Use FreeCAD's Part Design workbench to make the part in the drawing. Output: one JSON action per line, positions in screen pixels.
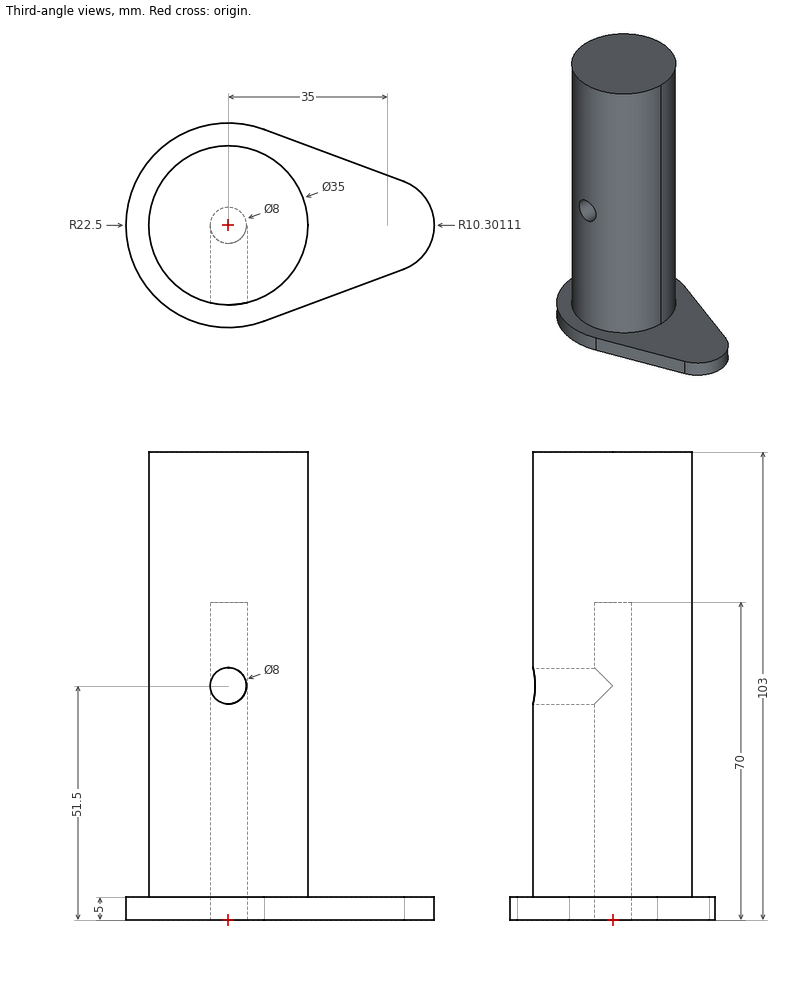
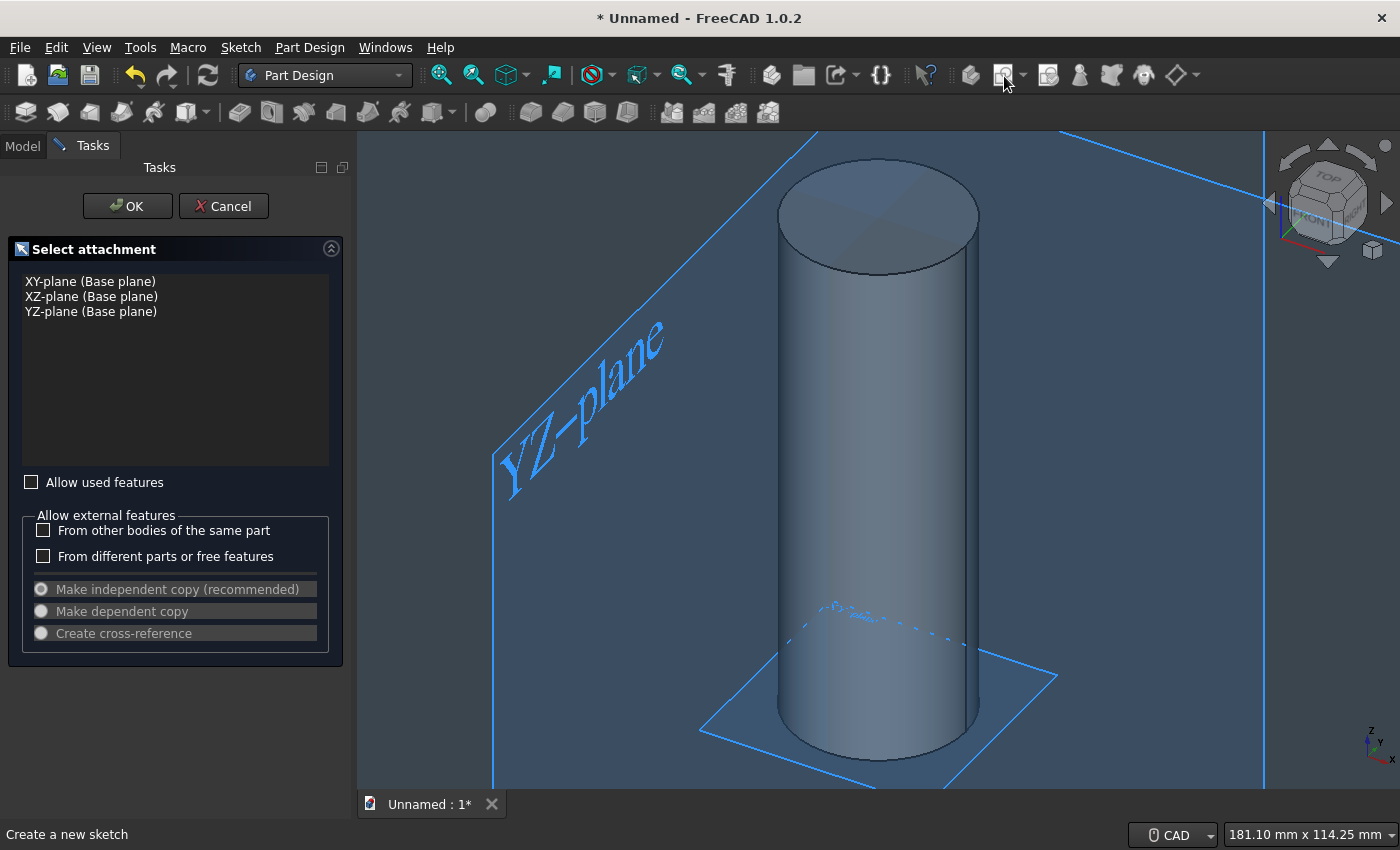
{"action": "left_click", "coordinate": [82, 282]}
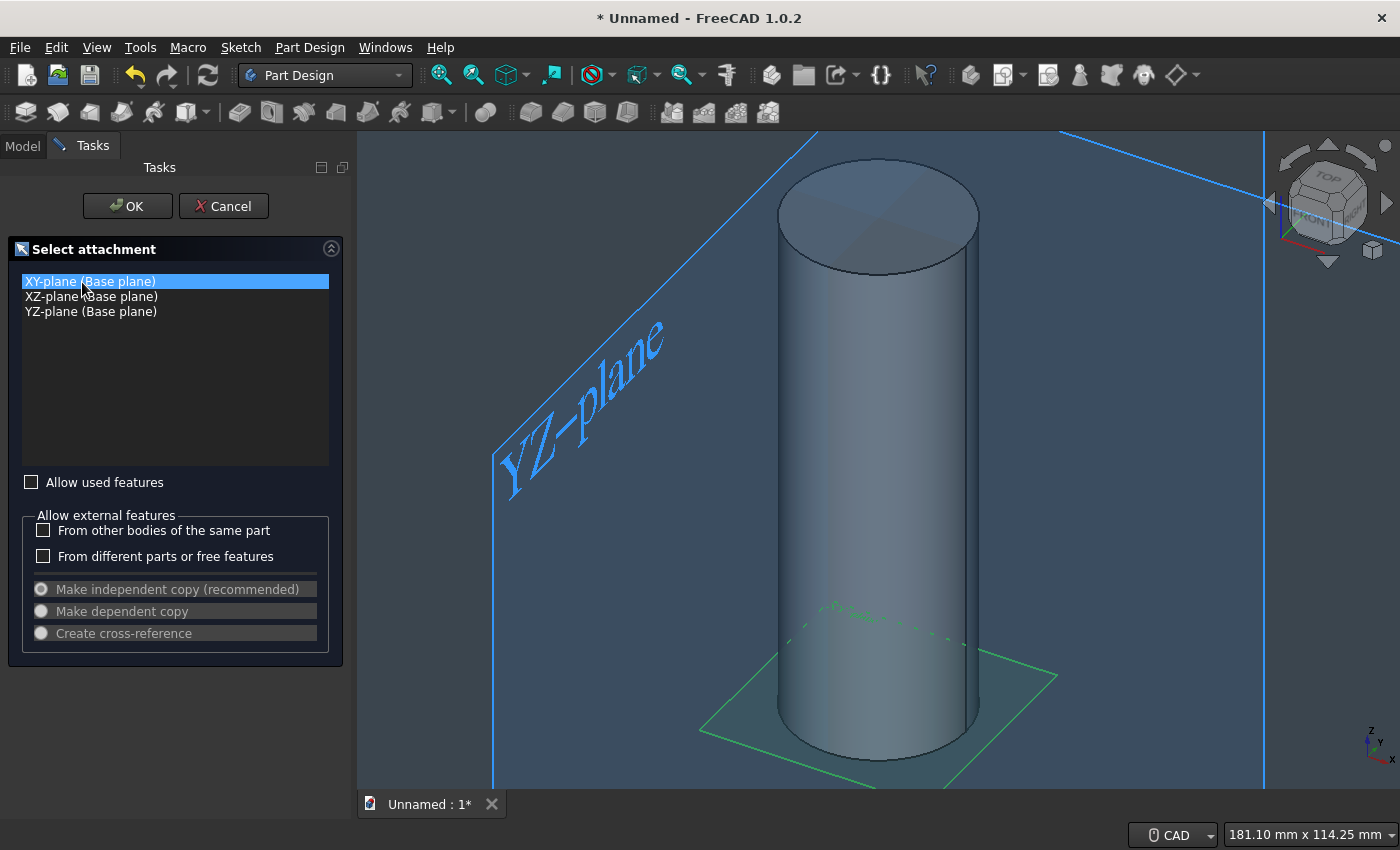
{"action": "left_click", "coordinate": [128, 206]}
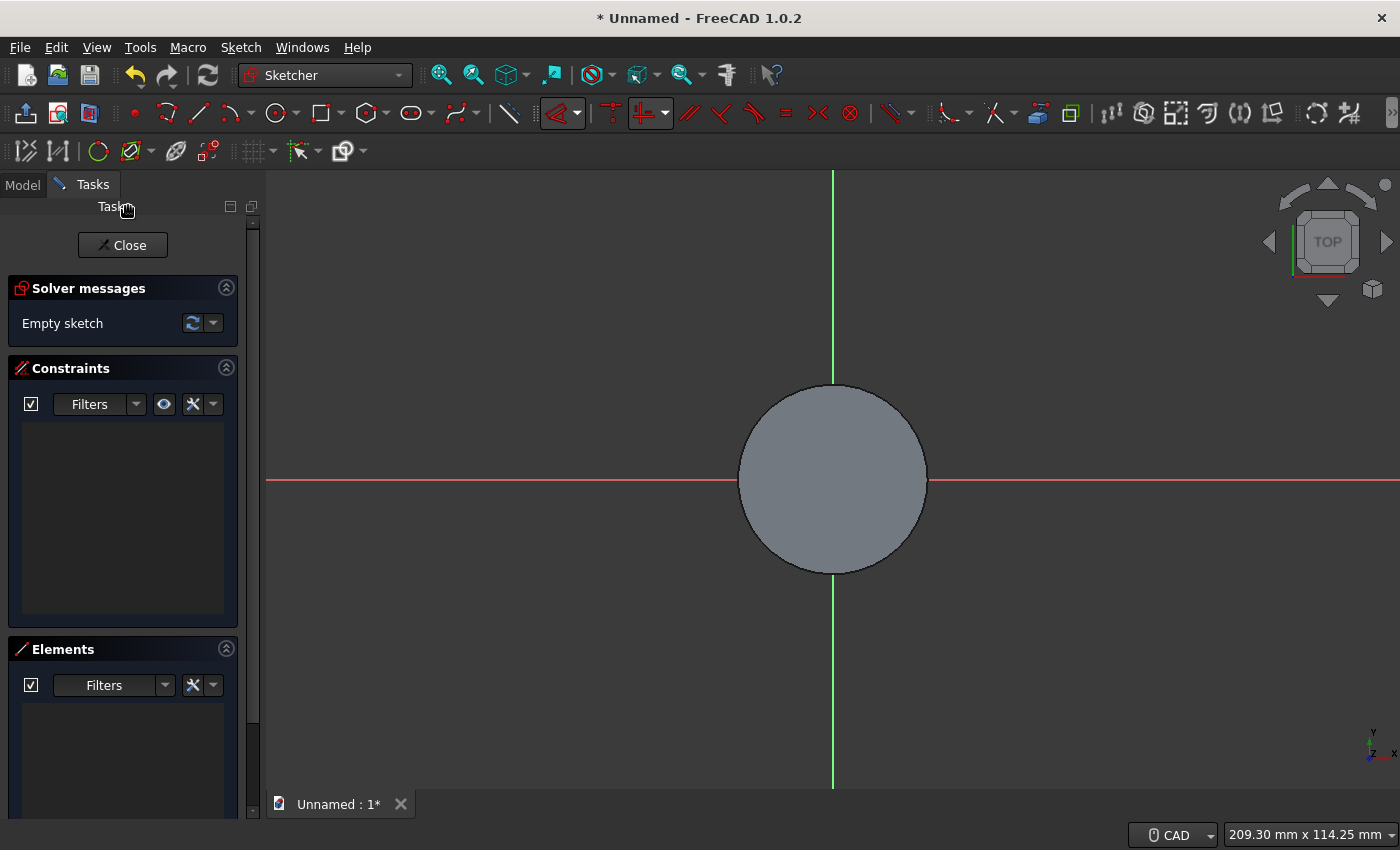
{"action": "left_click", "coordinate": [90, 114]}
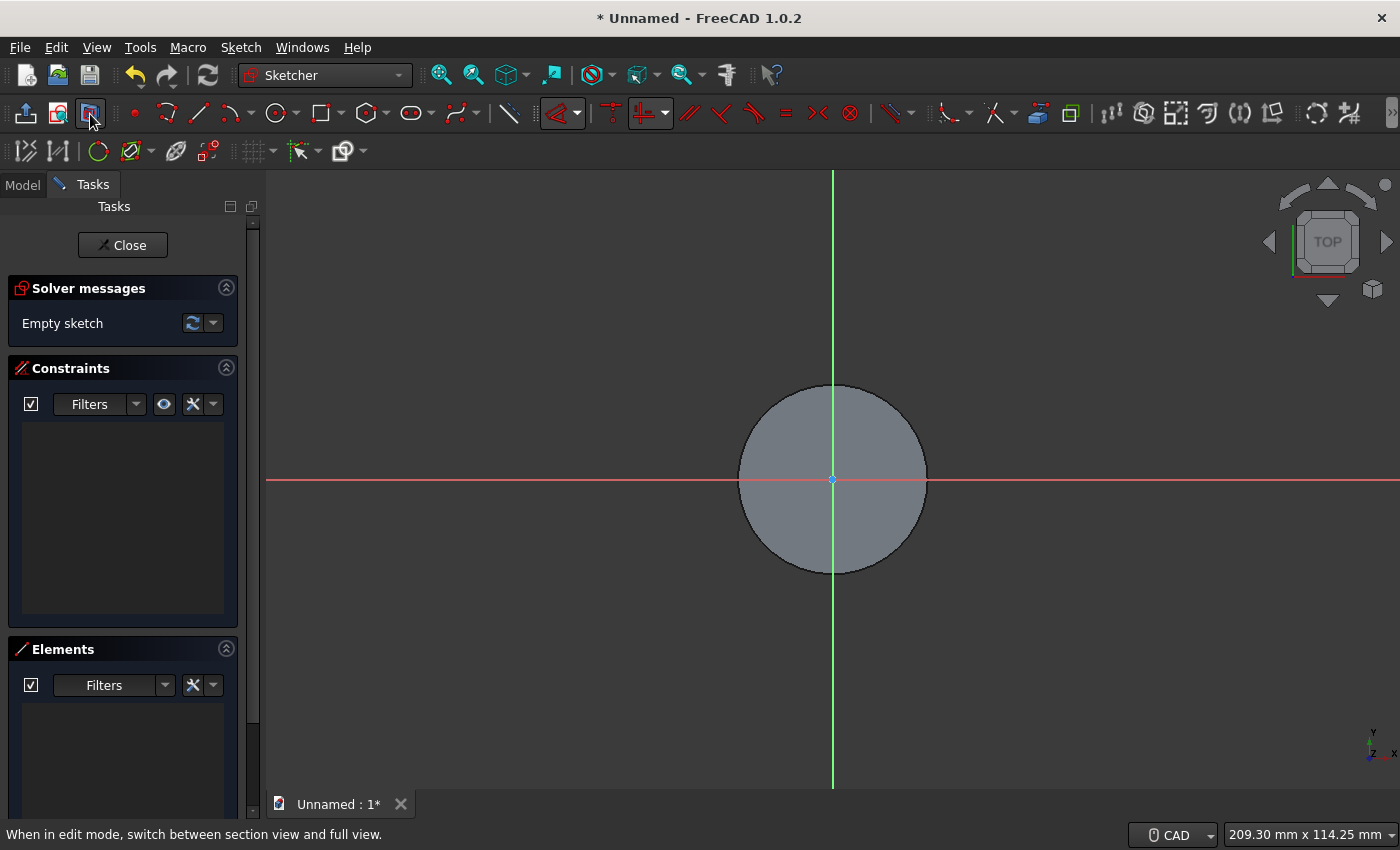
{"action": "scroll", "coordinate": [1053, 480], "scroll_direction": "up", "scroll_amount": 3}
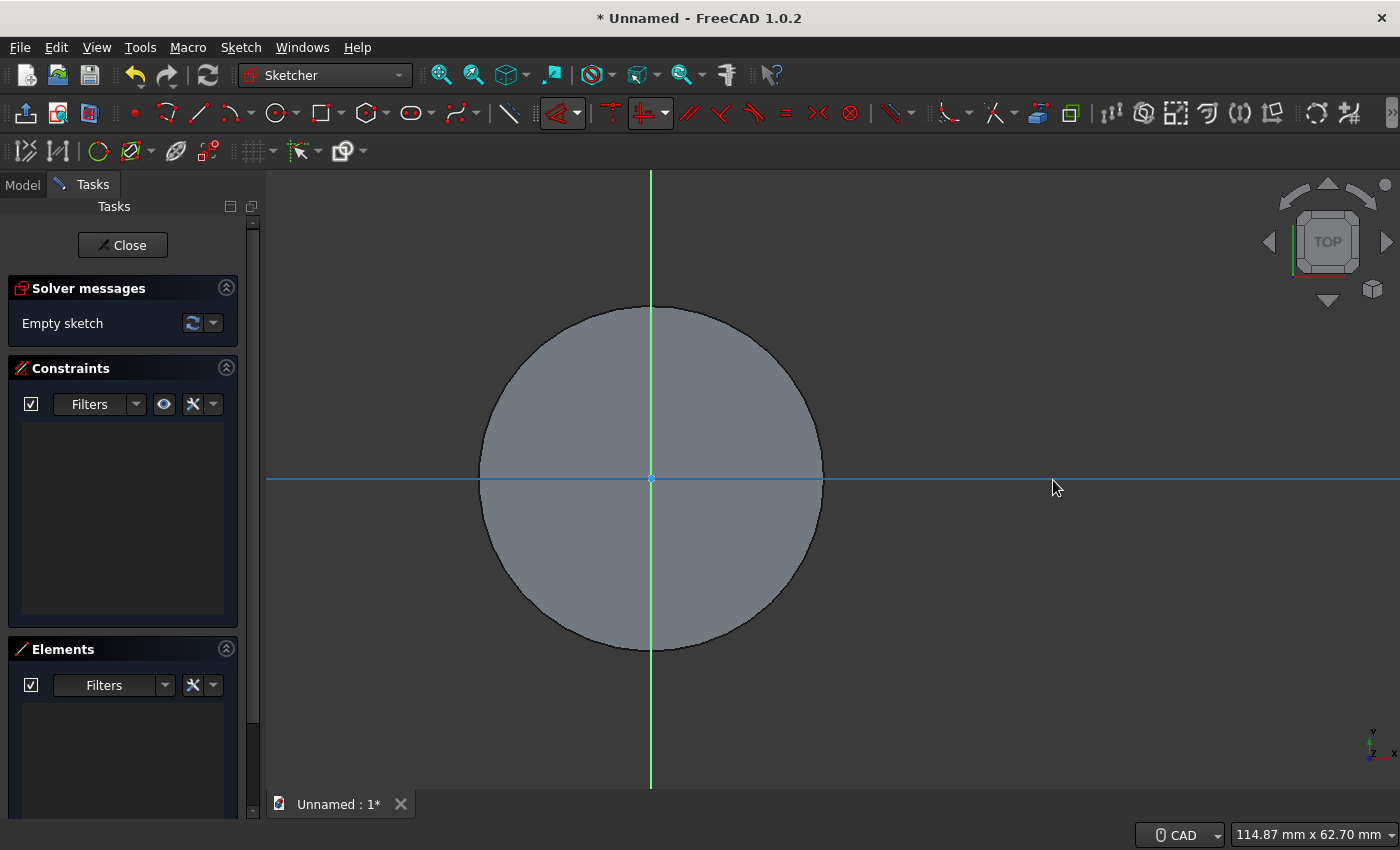
{"action": "left_click", "coordinate": [200, 114]}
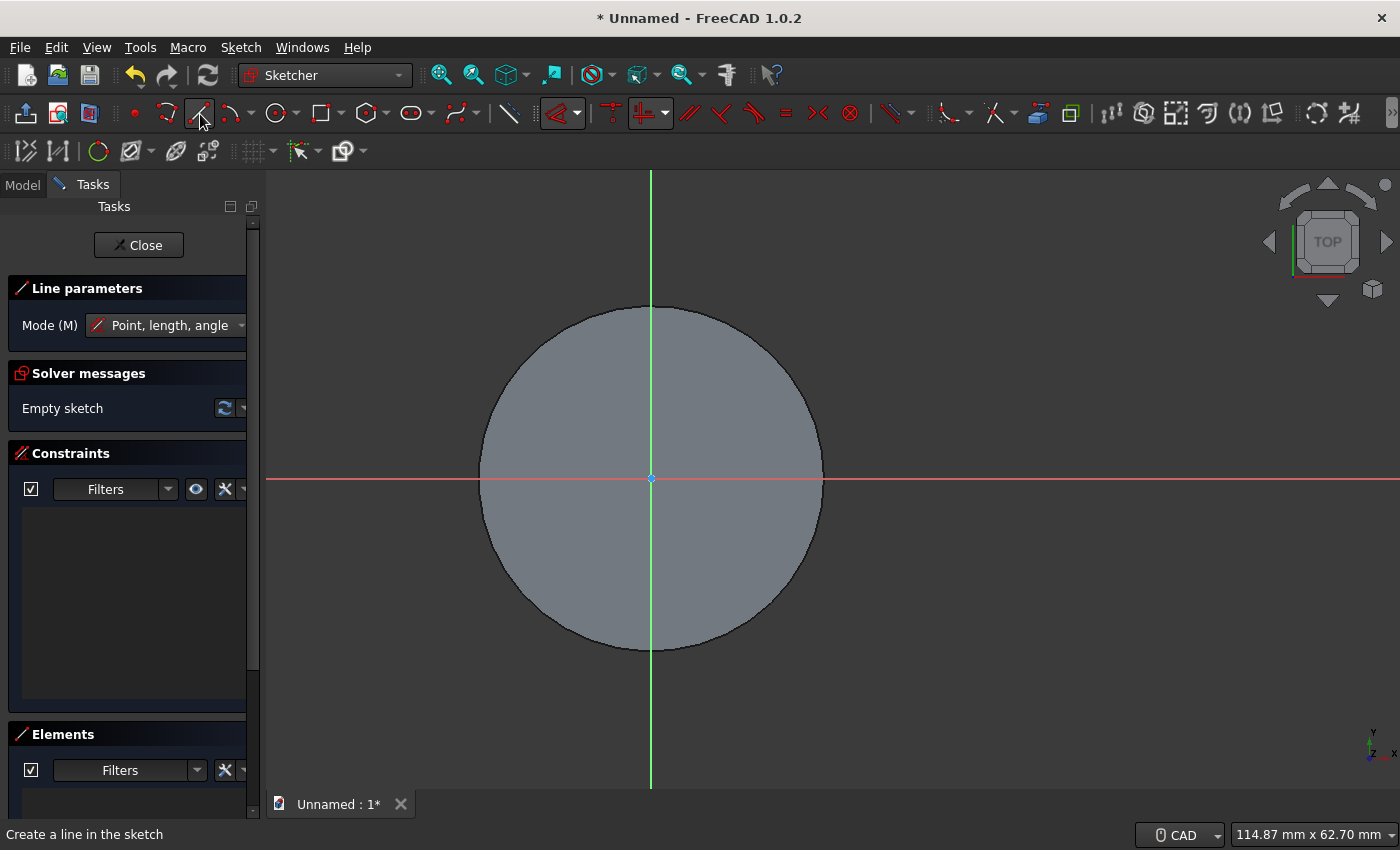
{"action": "left_click", "coordinate": [729, 270]}
{"action": "left_click", "coordinate": [1032, 383]}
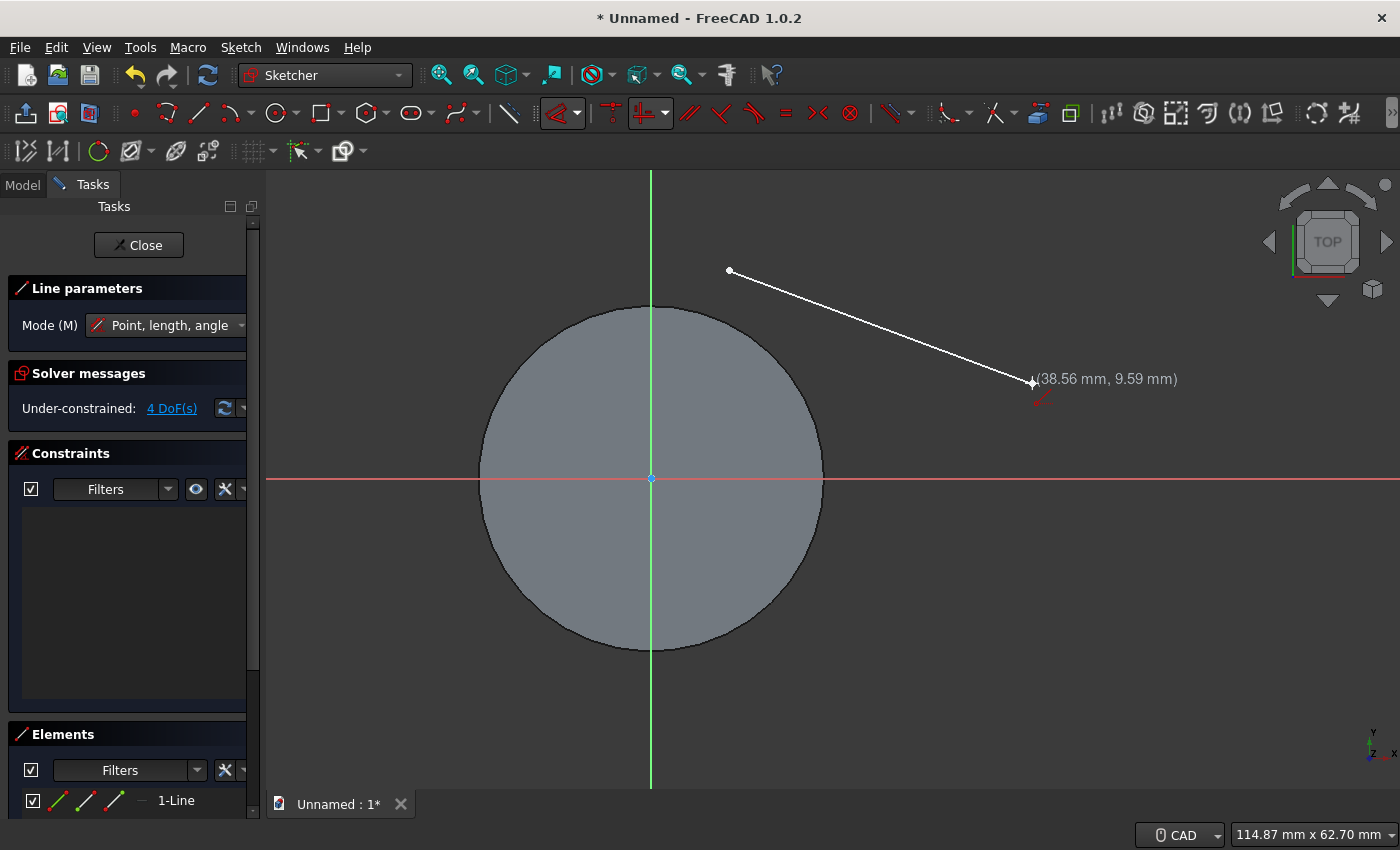
{"action": "left_click", "coordinate": [1032, 574]}
{"action": "left_click", "coordinate": [729, 687]}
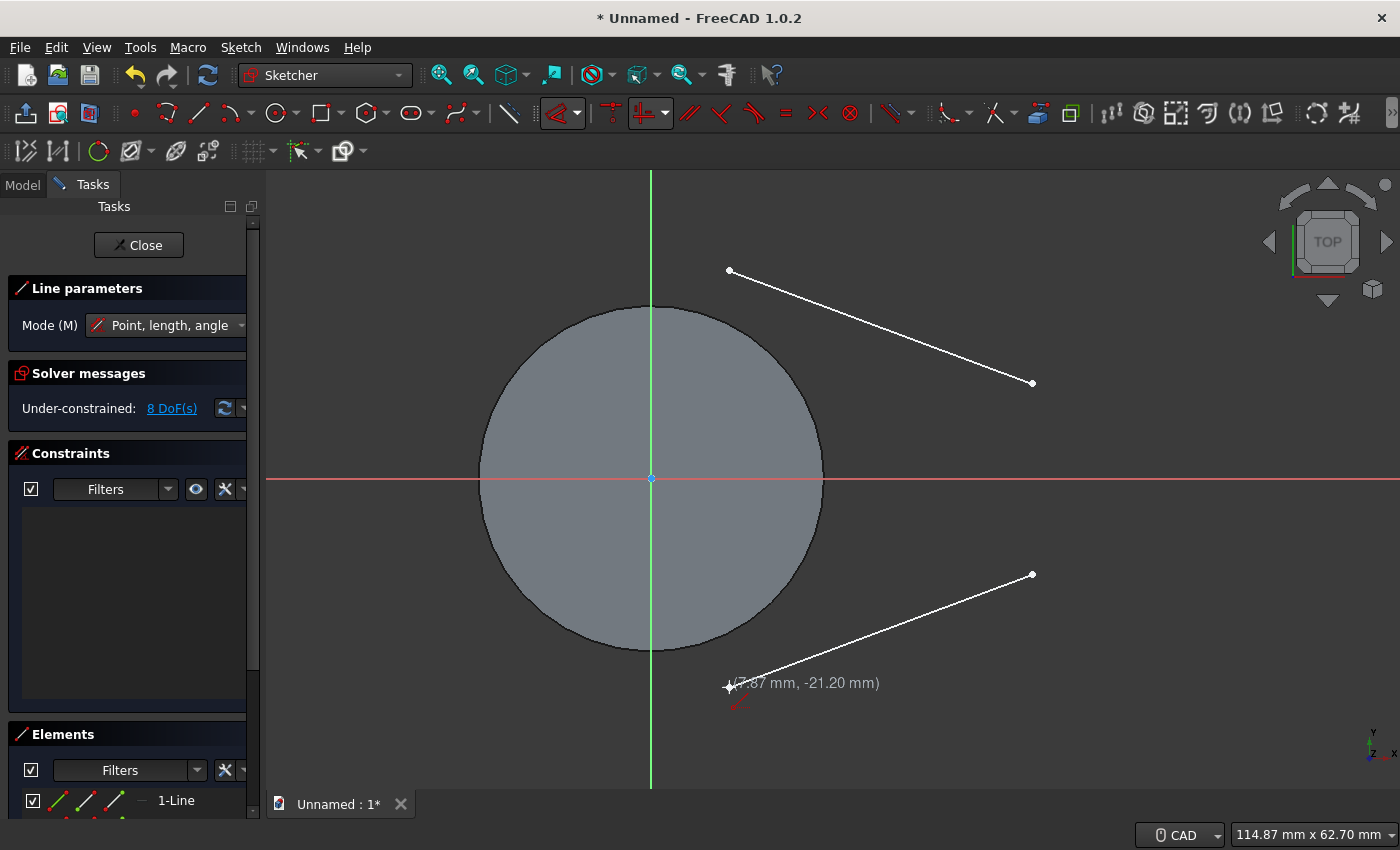
{"action": "key", "text": "g 3 a"}